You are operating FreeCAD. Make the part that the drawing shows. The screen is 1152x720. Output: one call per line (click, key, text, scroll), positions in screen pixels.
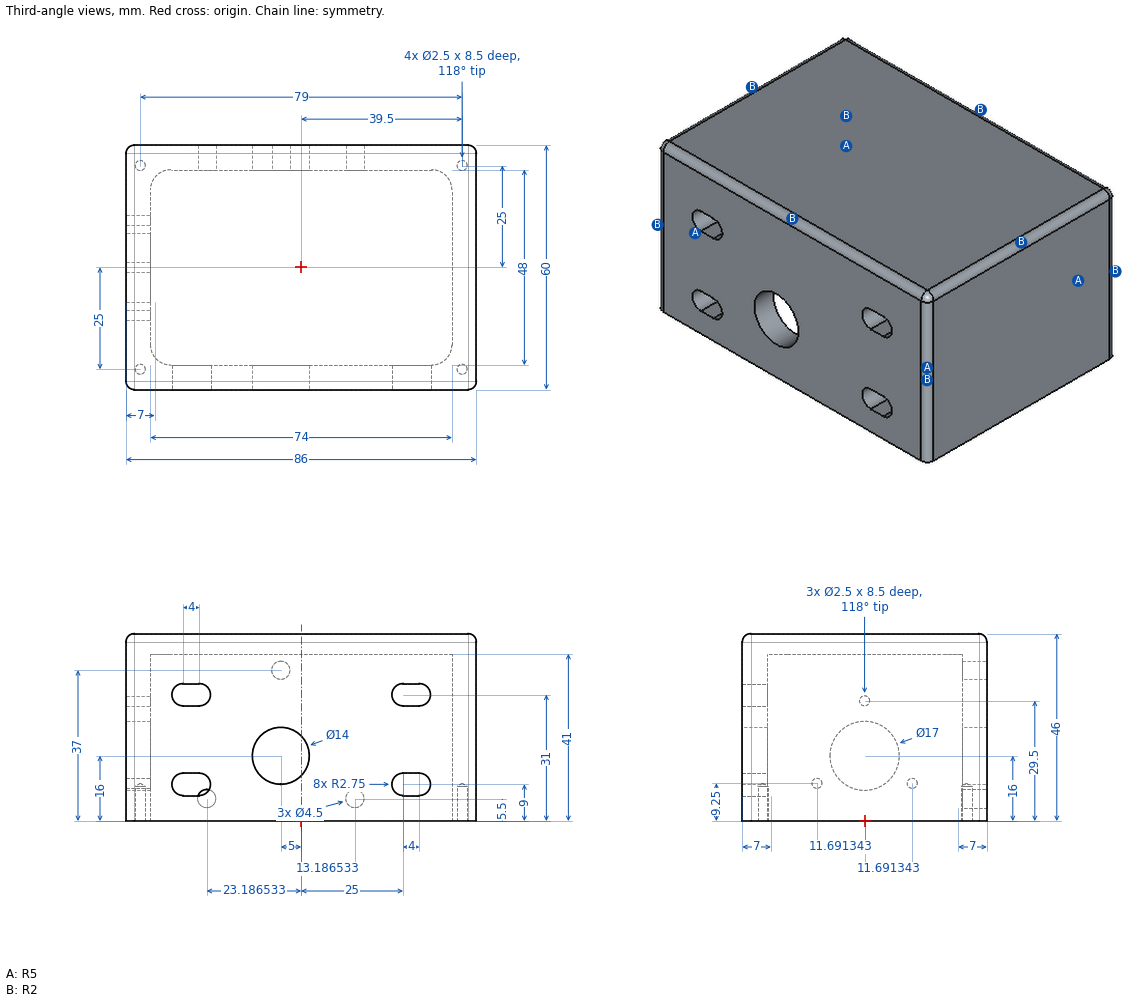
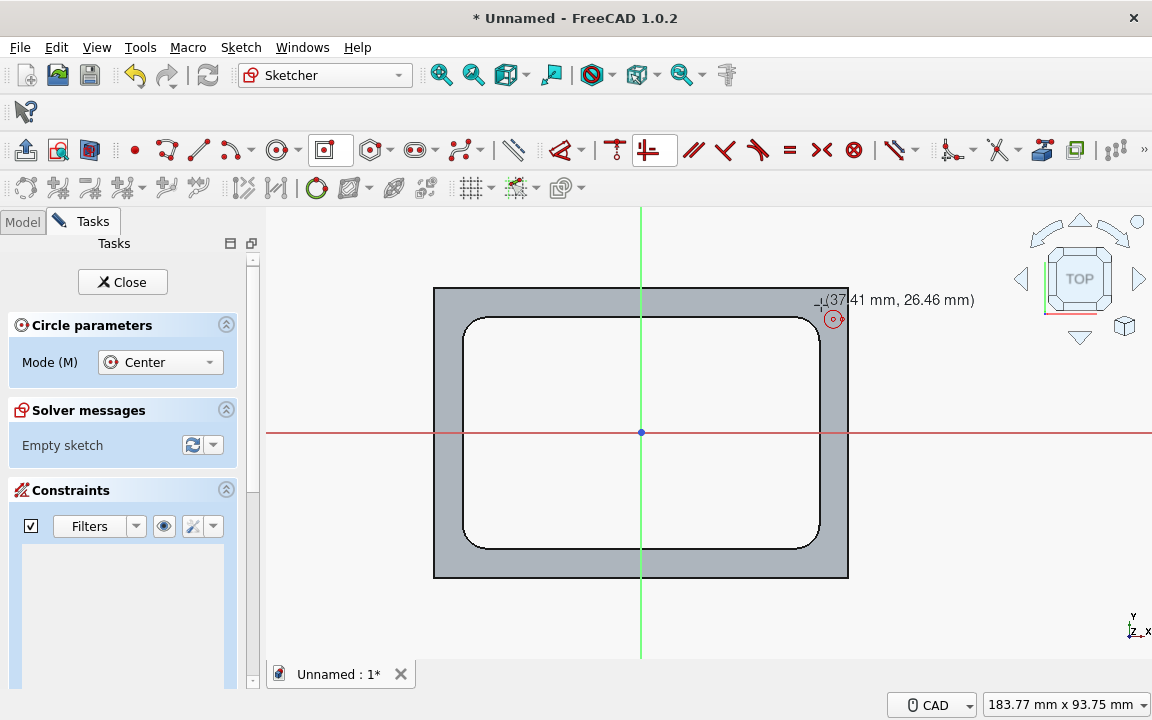
click(832, 312)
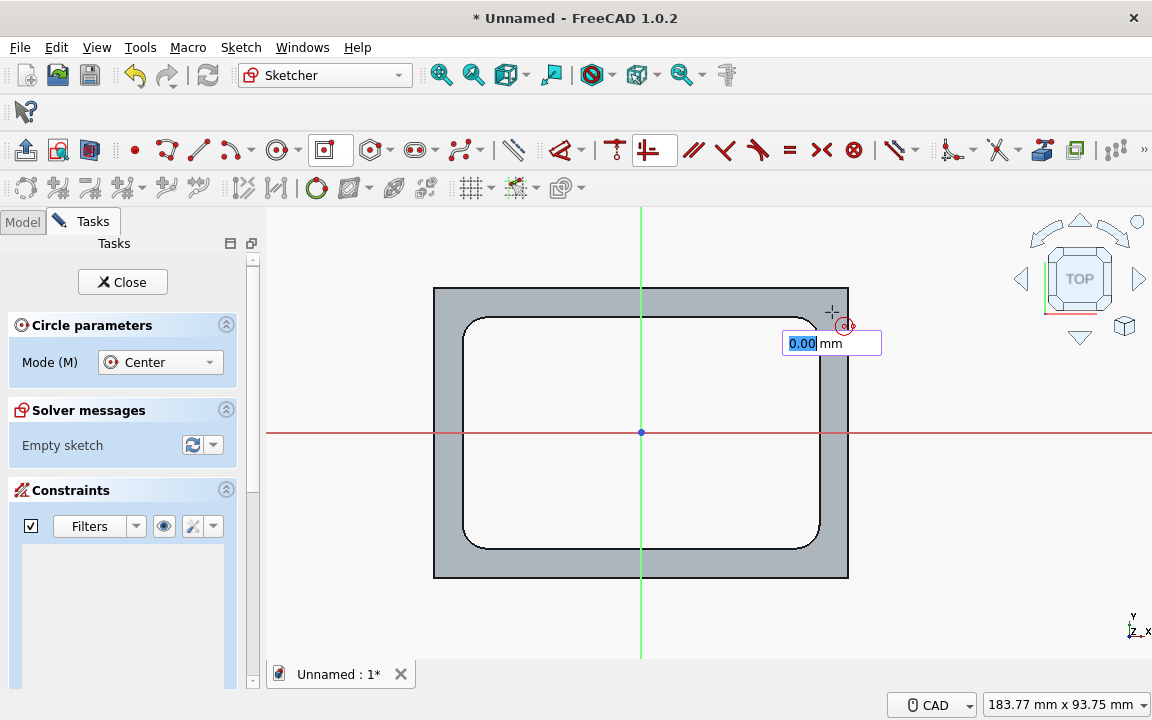
scroll(836, 308, up, 5)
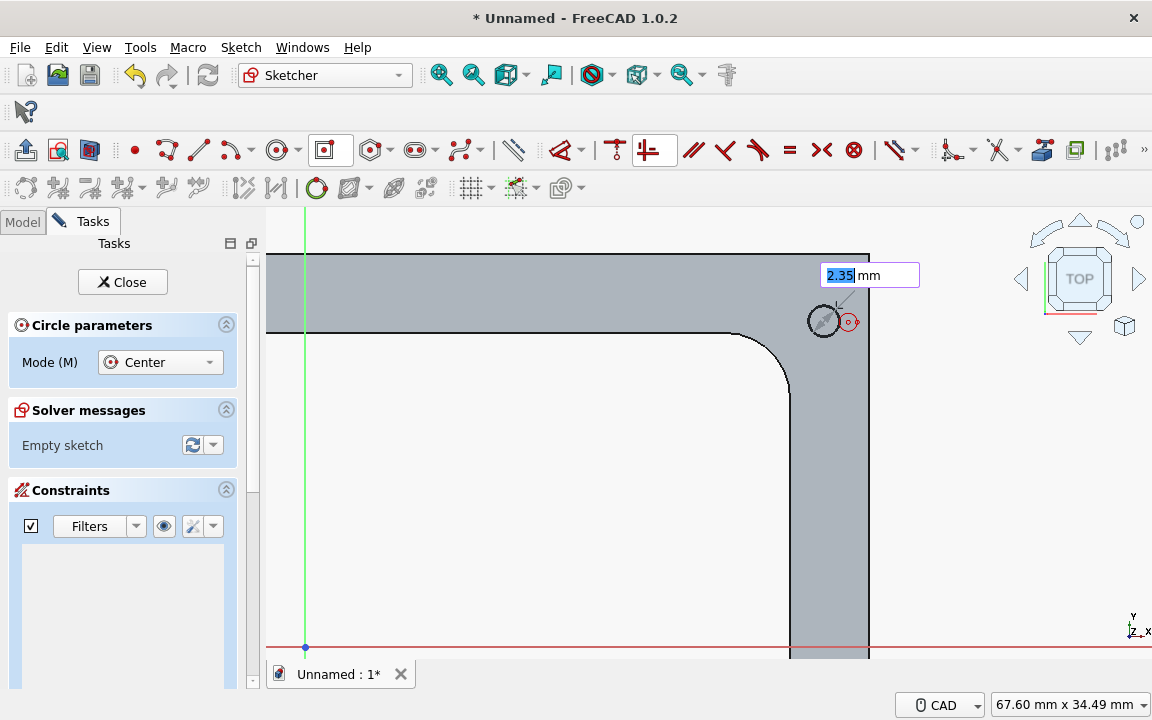
click(834, 308)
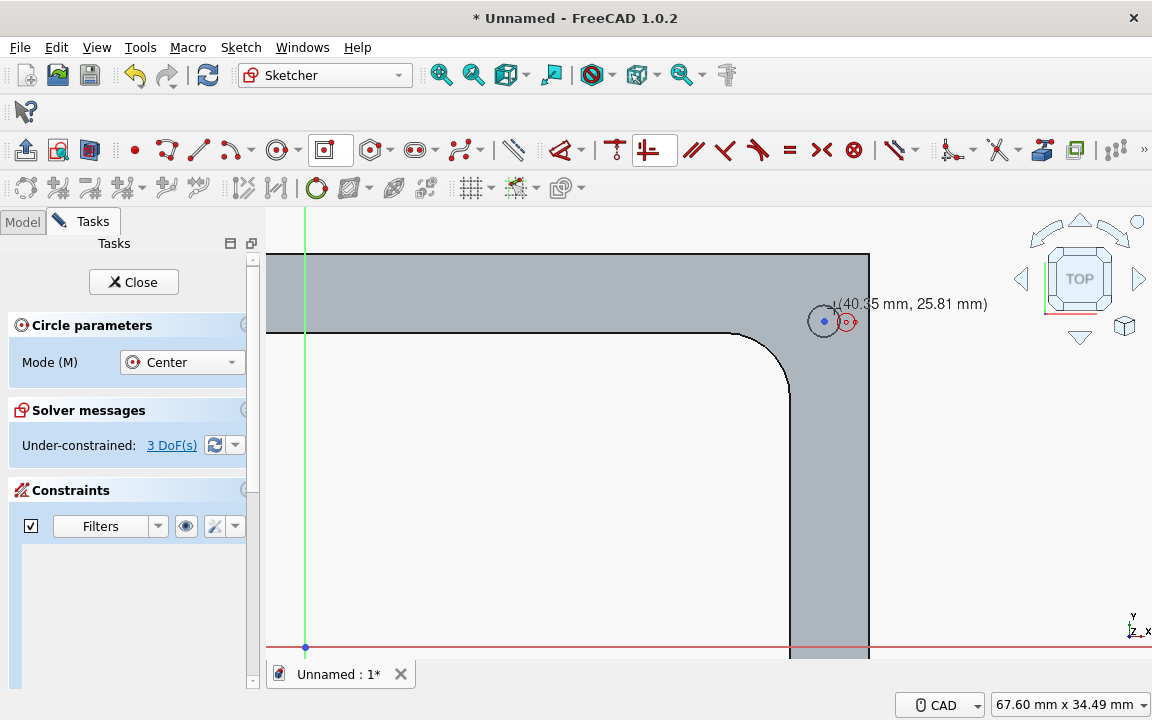
scroll(836, 308, down, 5)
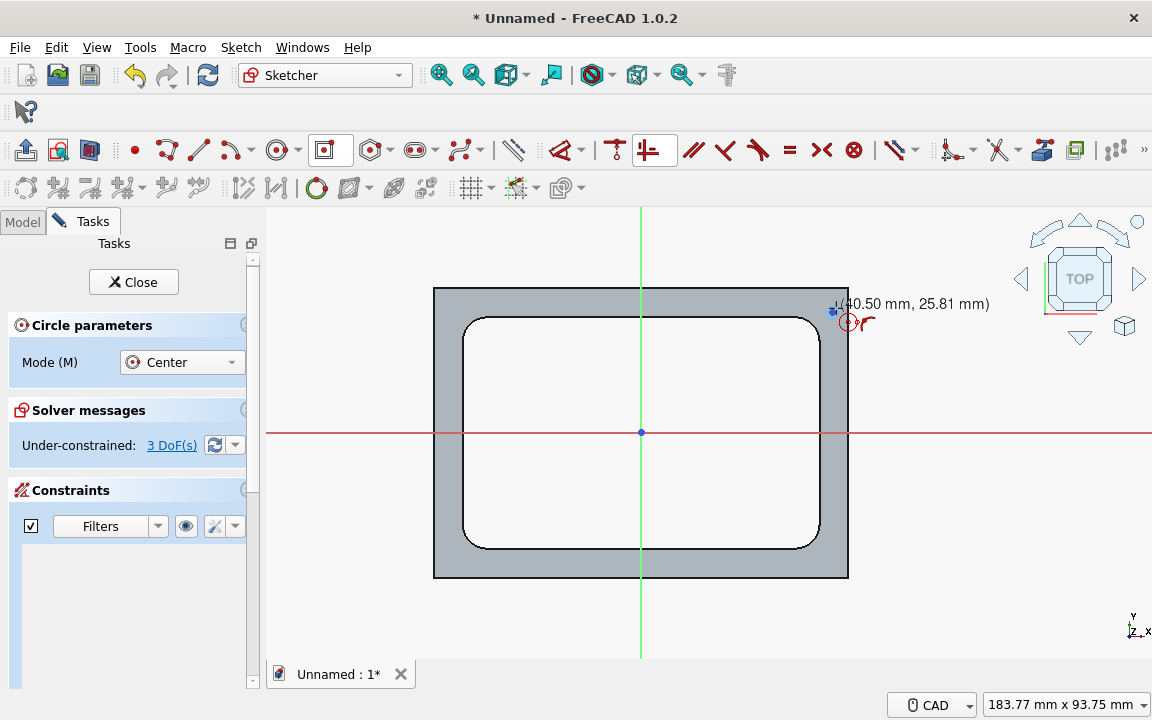
scroll(451, 312, up, 7)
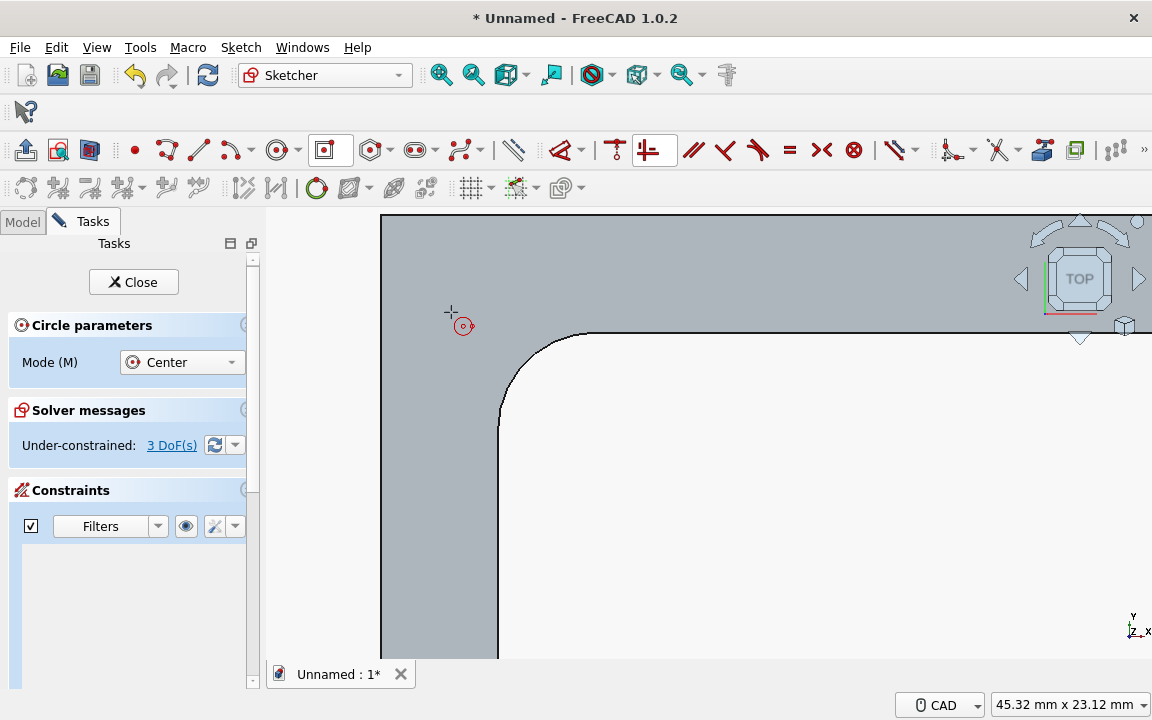
scroll(450, 312, down, 7)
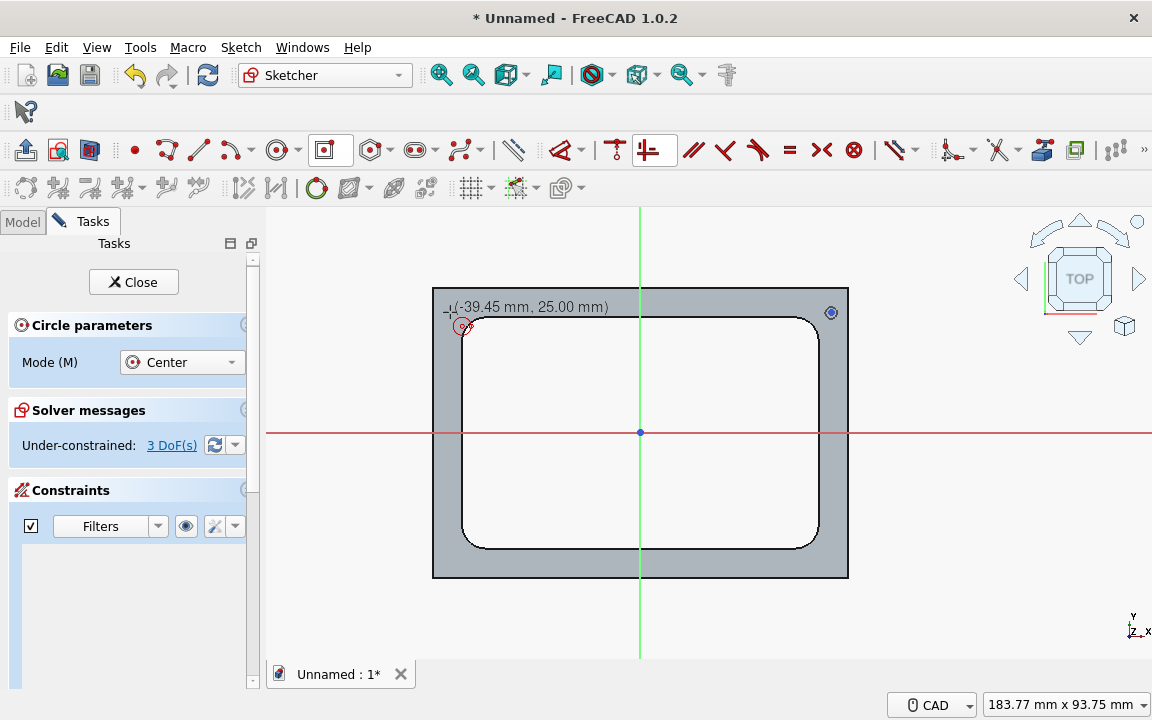
click(450, 312)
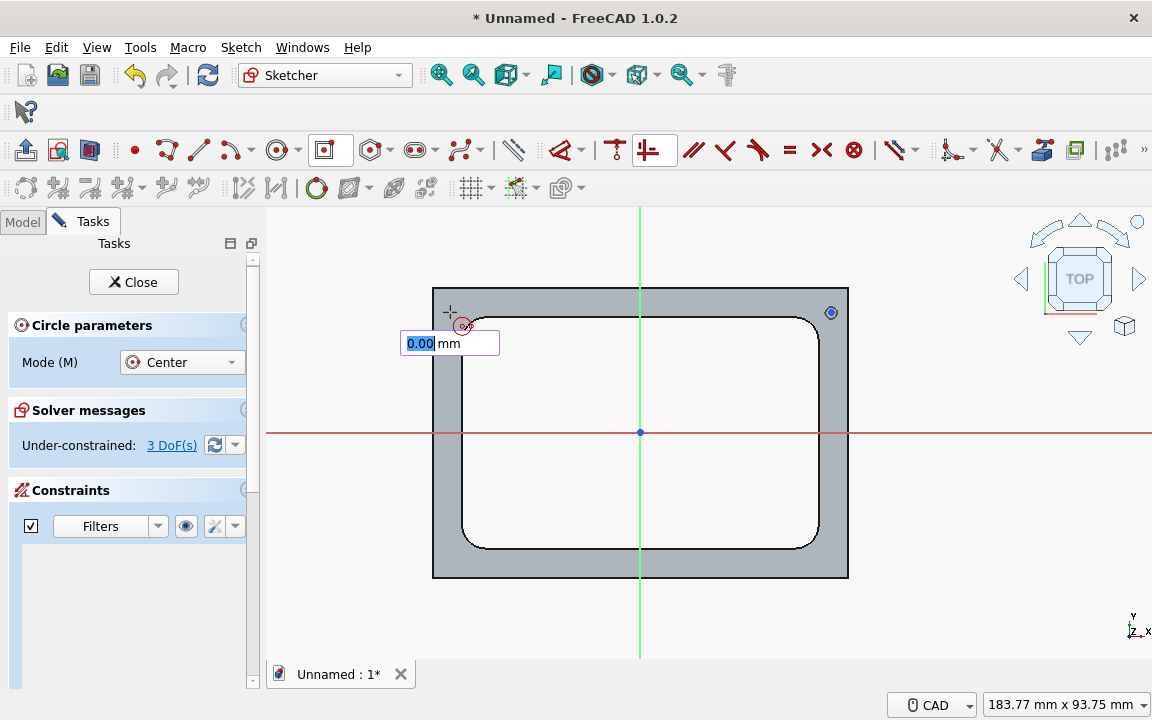
scroll(454, 308, up, 5)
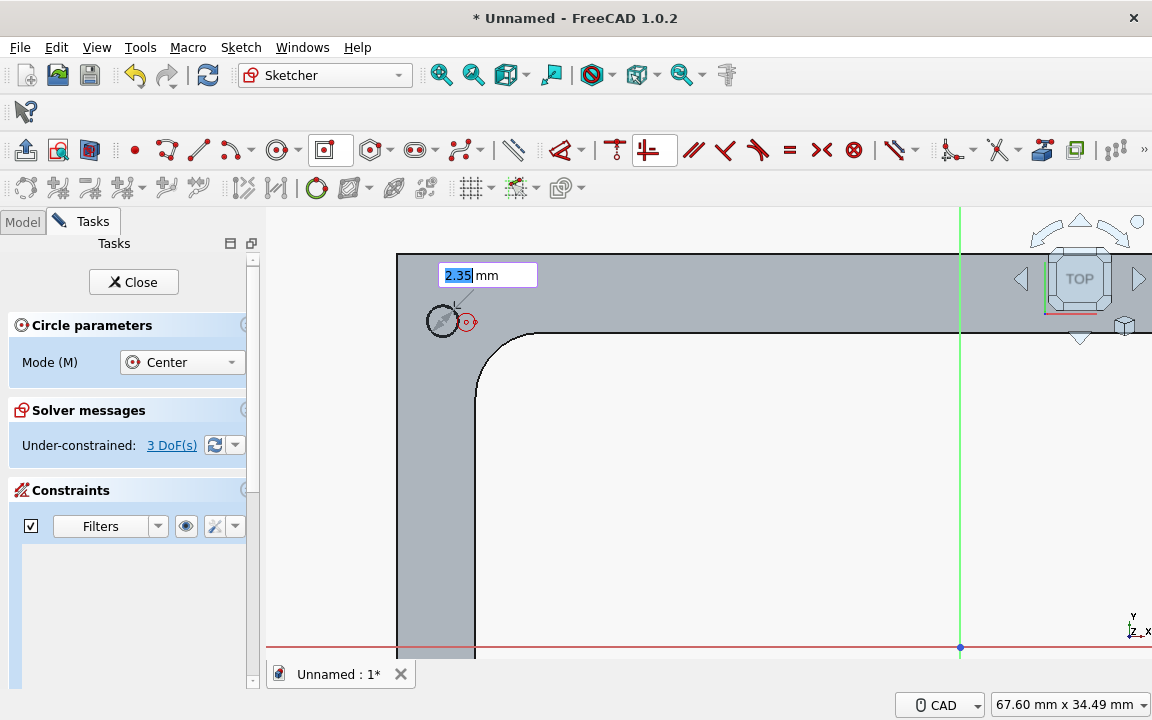
click(454, 308)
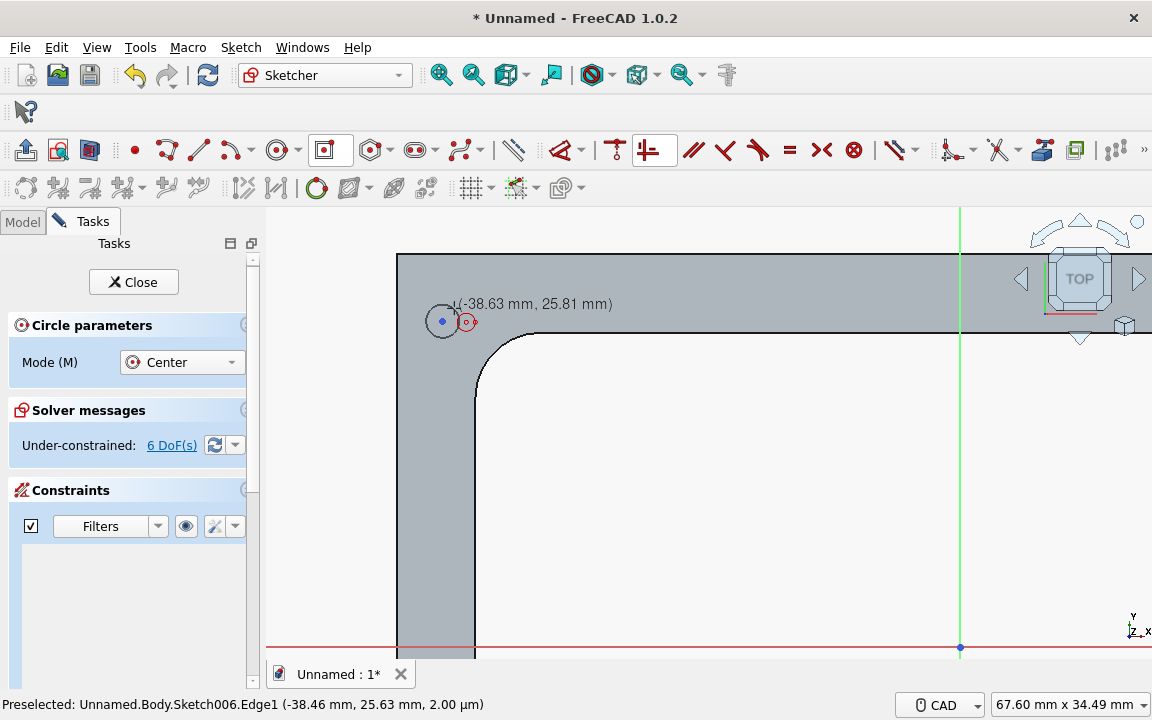
scroll(454, 308, down, 5)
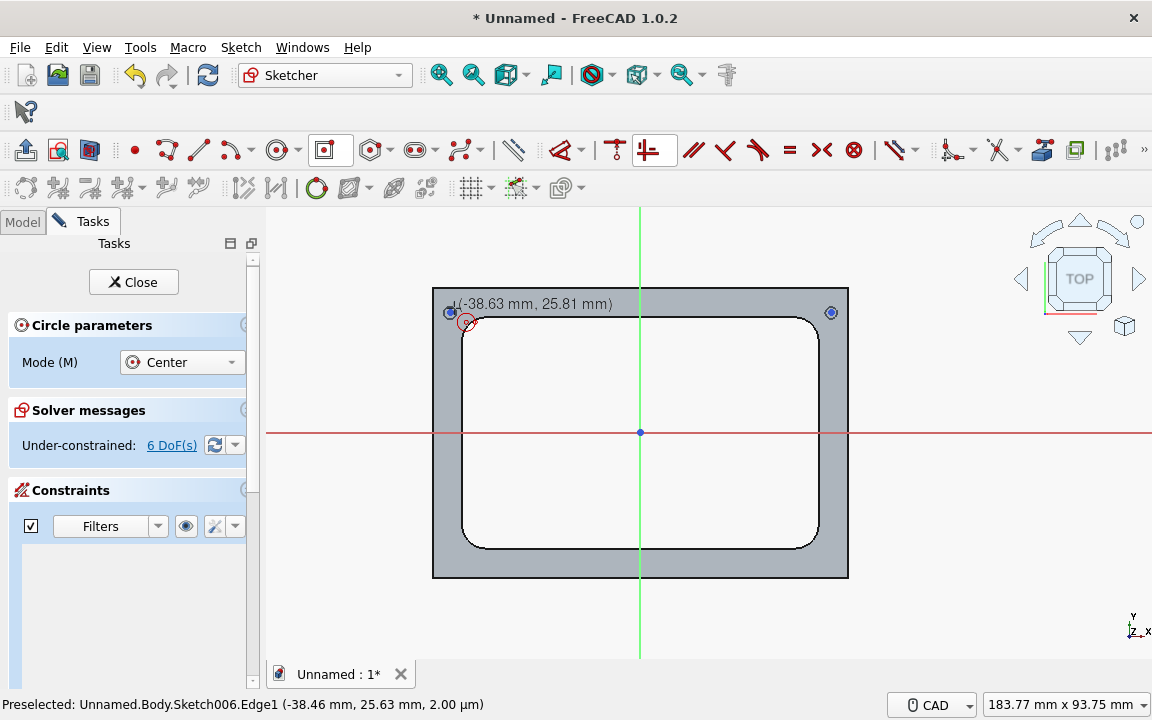
scroll(450, 553, up, 7)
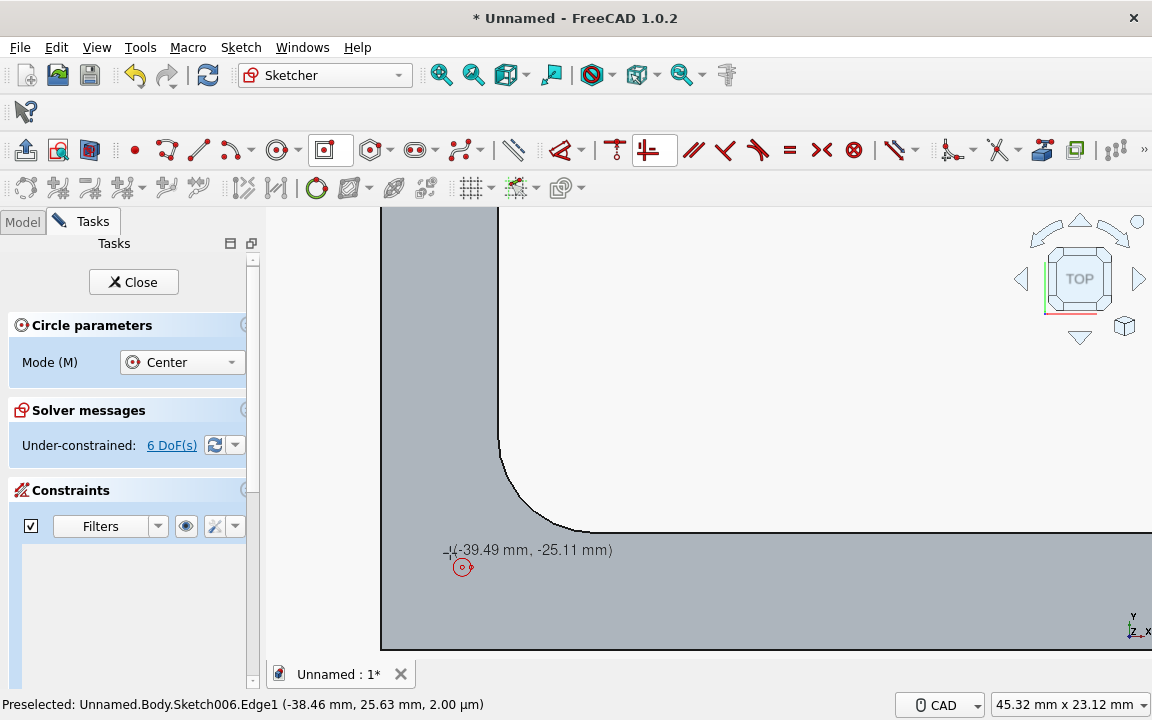
scroll(450, 554, down, 7)